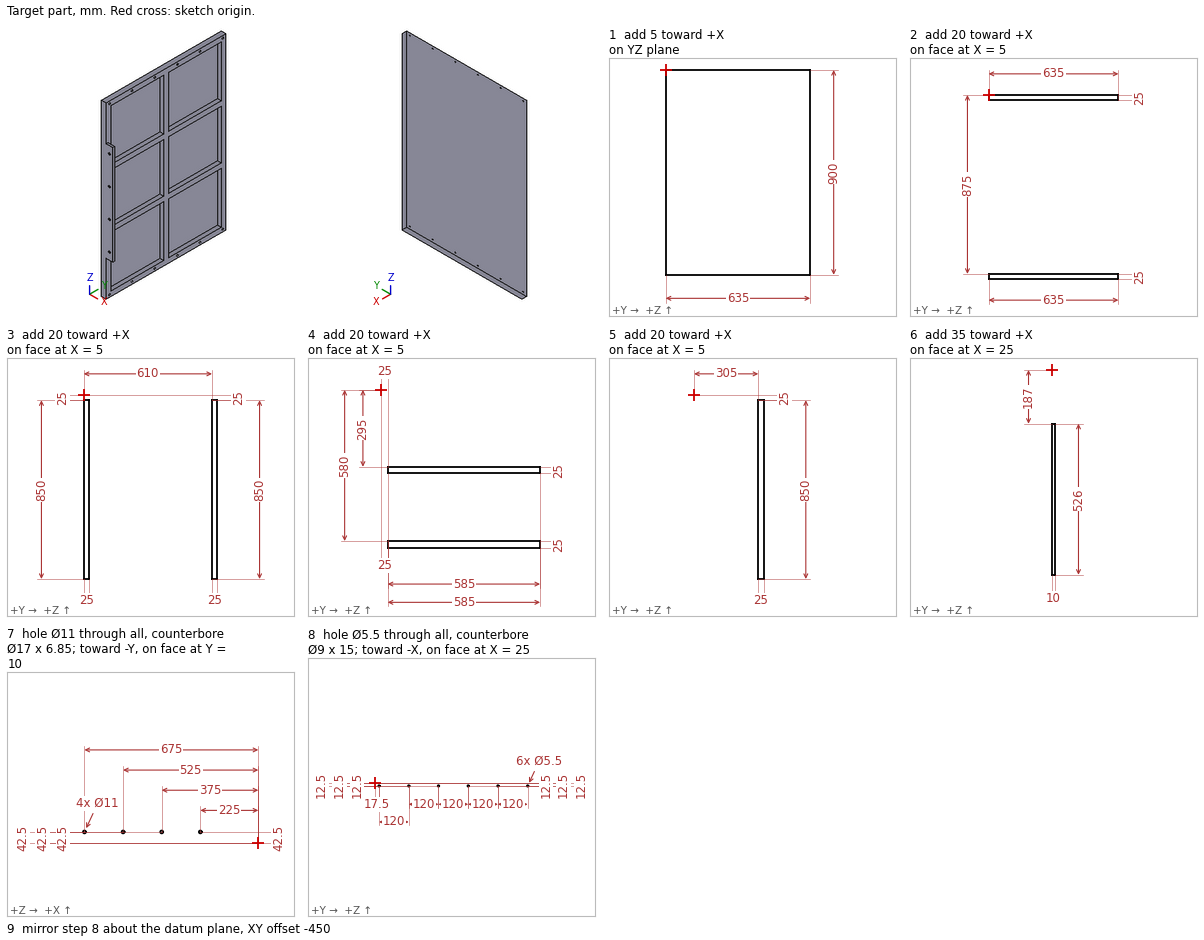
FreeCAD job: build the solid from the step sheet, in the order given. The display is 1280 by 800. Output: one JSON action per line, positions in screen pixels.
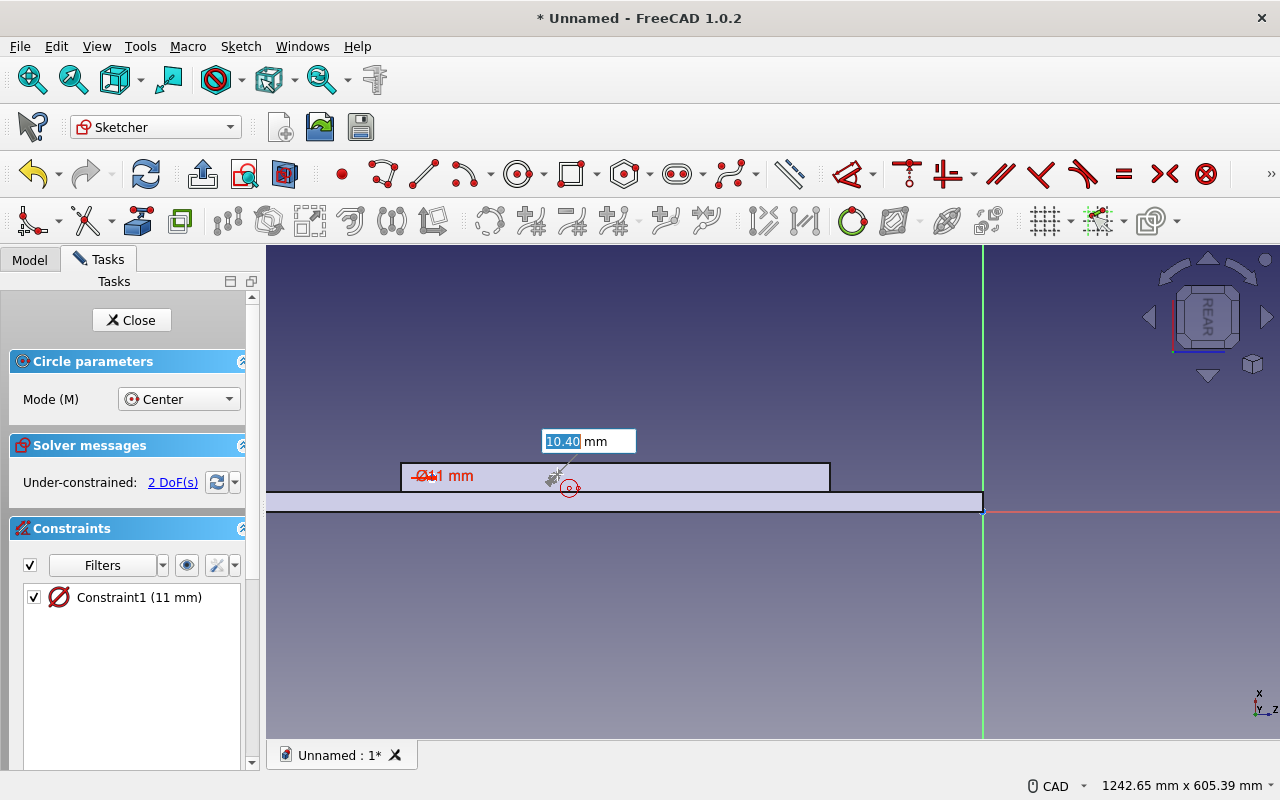
{"action": "type", "text": "11"}
{"action": "key", "text": "Return"}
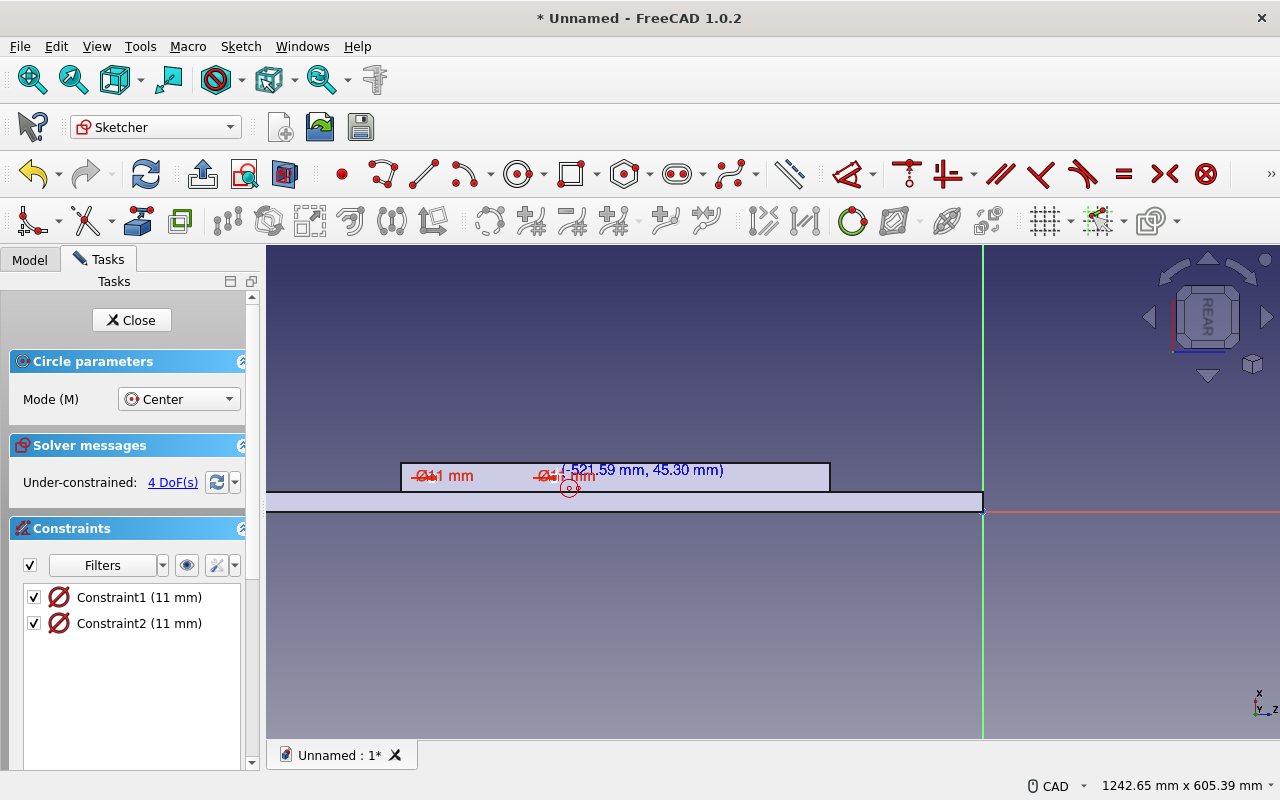
{"action": "scroll", "coordinate": [677, 477], "scroll_direction": "up", "scroll_amount": 9}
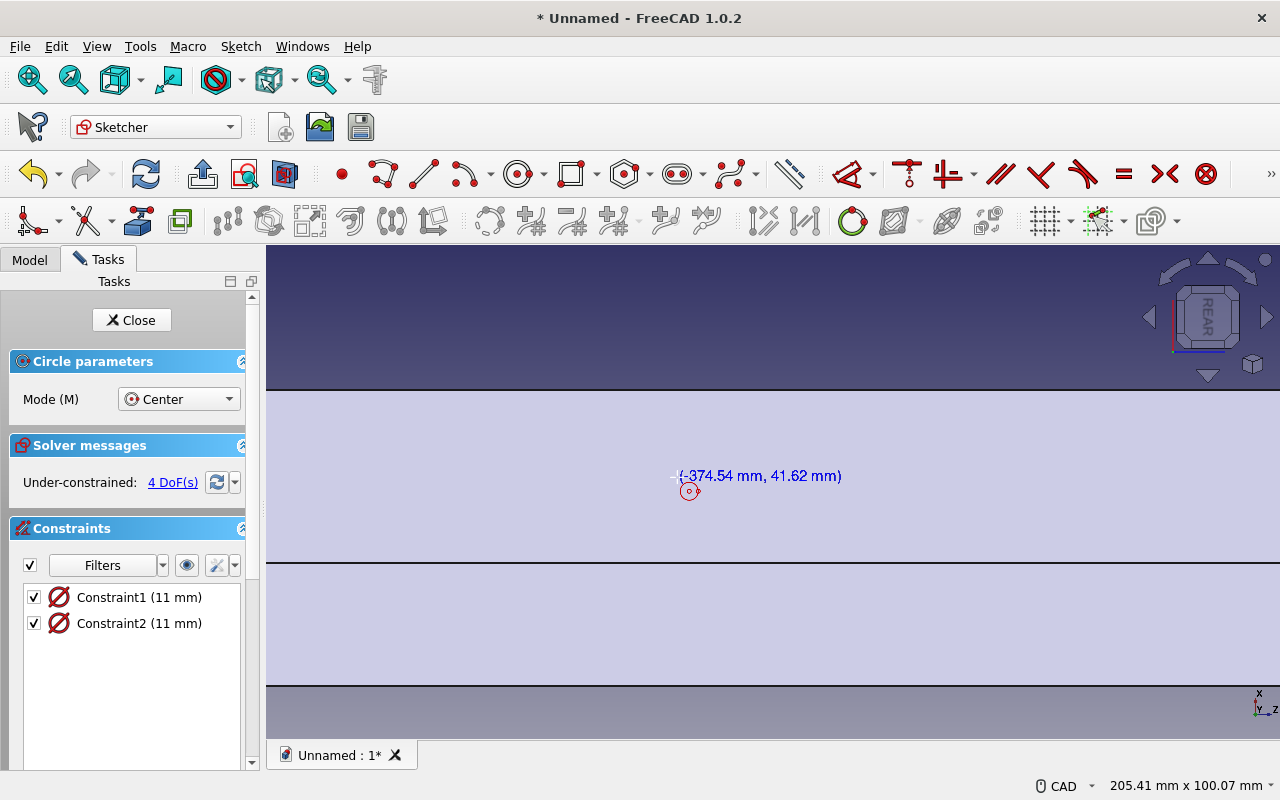
{"action": "scroll", "coordinate": [677, 477], "scroll_direction": "down", "scroll_amount": 9}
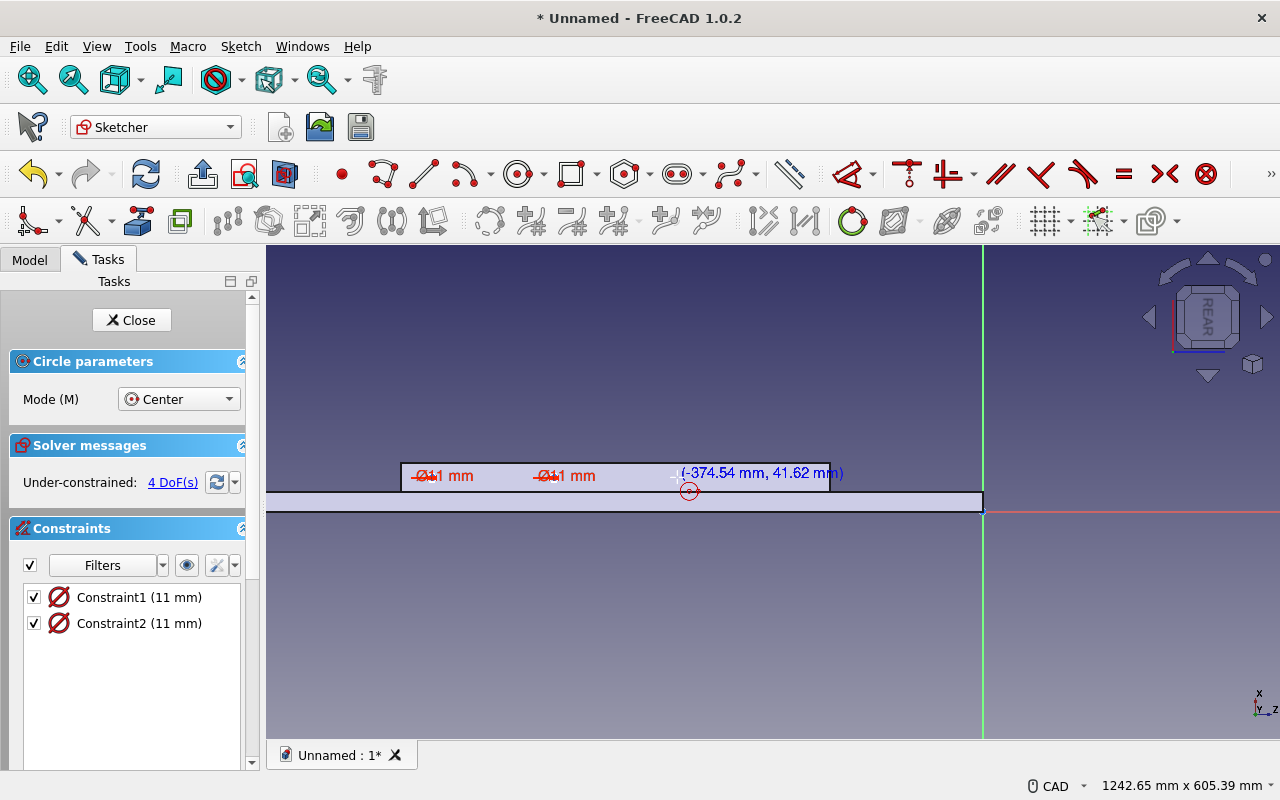
{"action": "left_click", "coordinate": [677, 477]}
{"action": "mouse_move", "coordinate": [680, 474]}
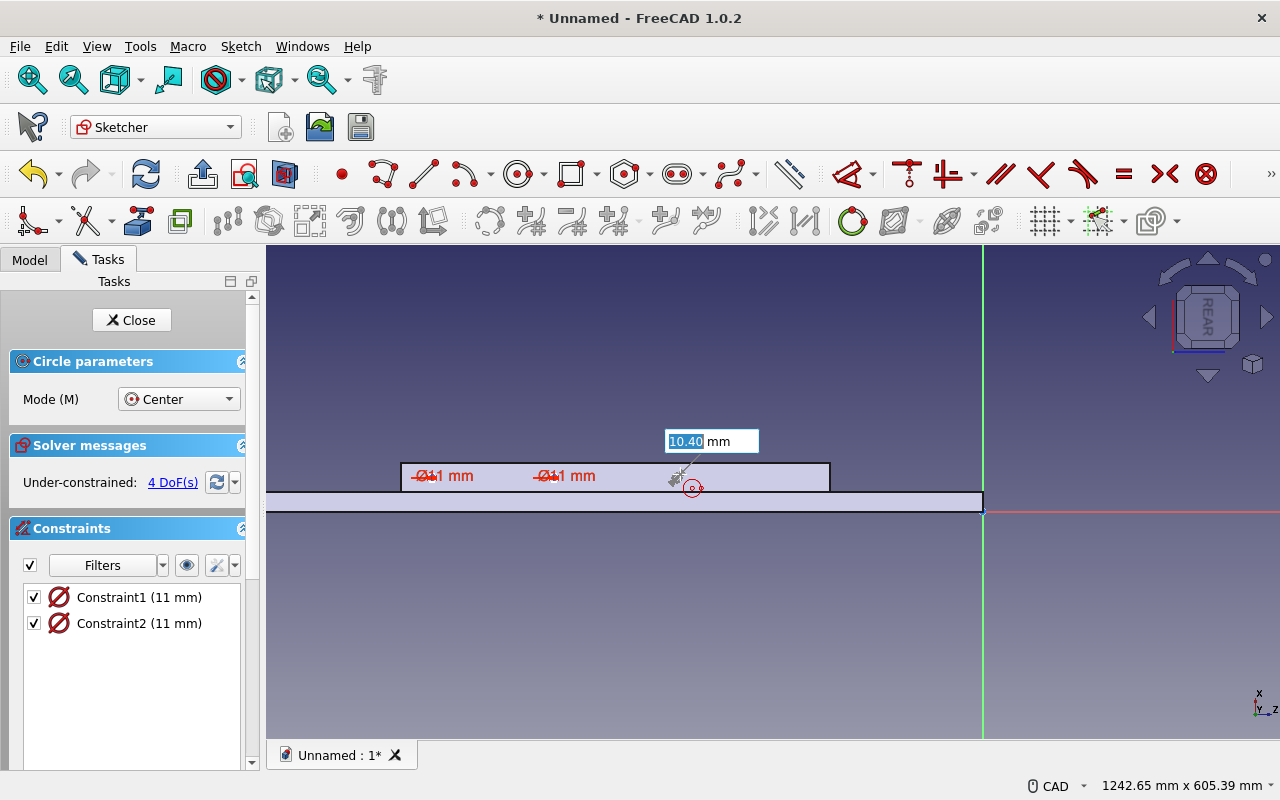
{"action": "type", "text": "11"}
{"action": "key", "text": "Return"}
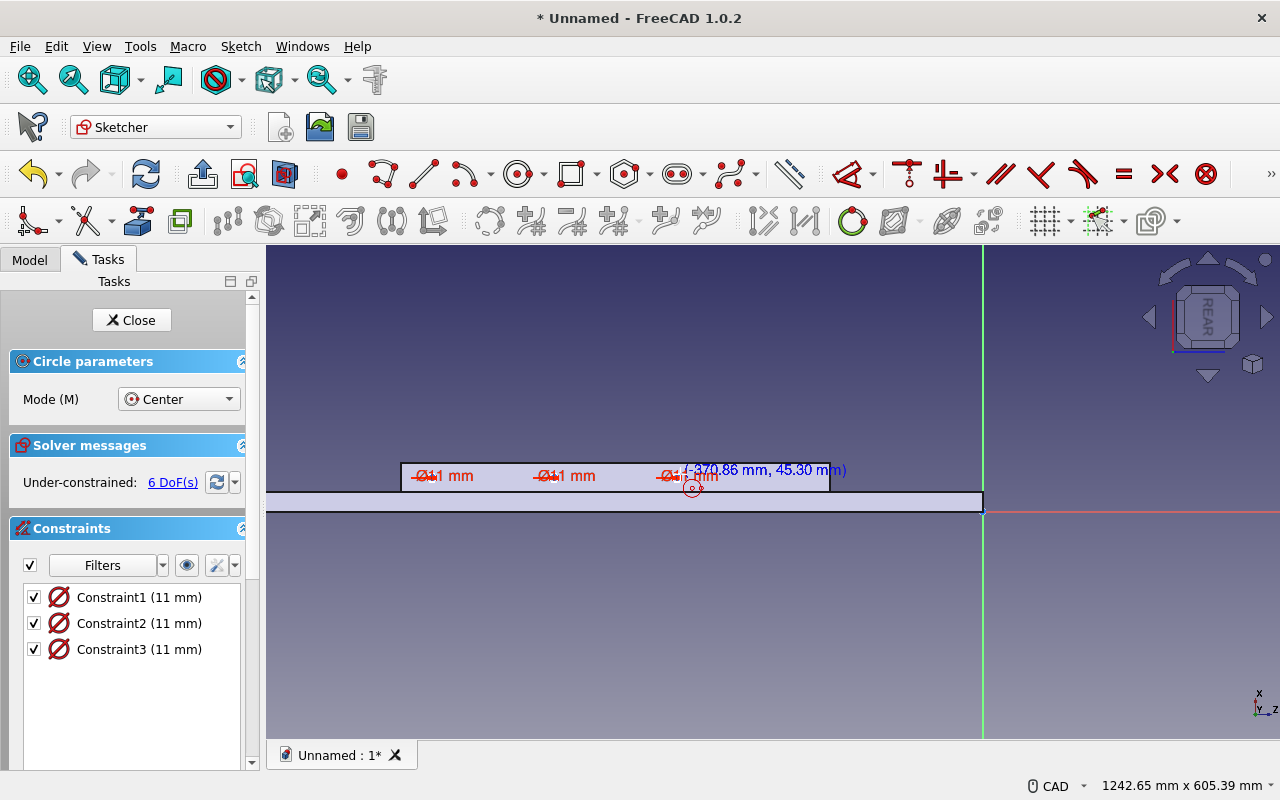
{"action": "scroll", "coordinate": [799, 477], "scroll_direction": "up", "scroll_amount": 9}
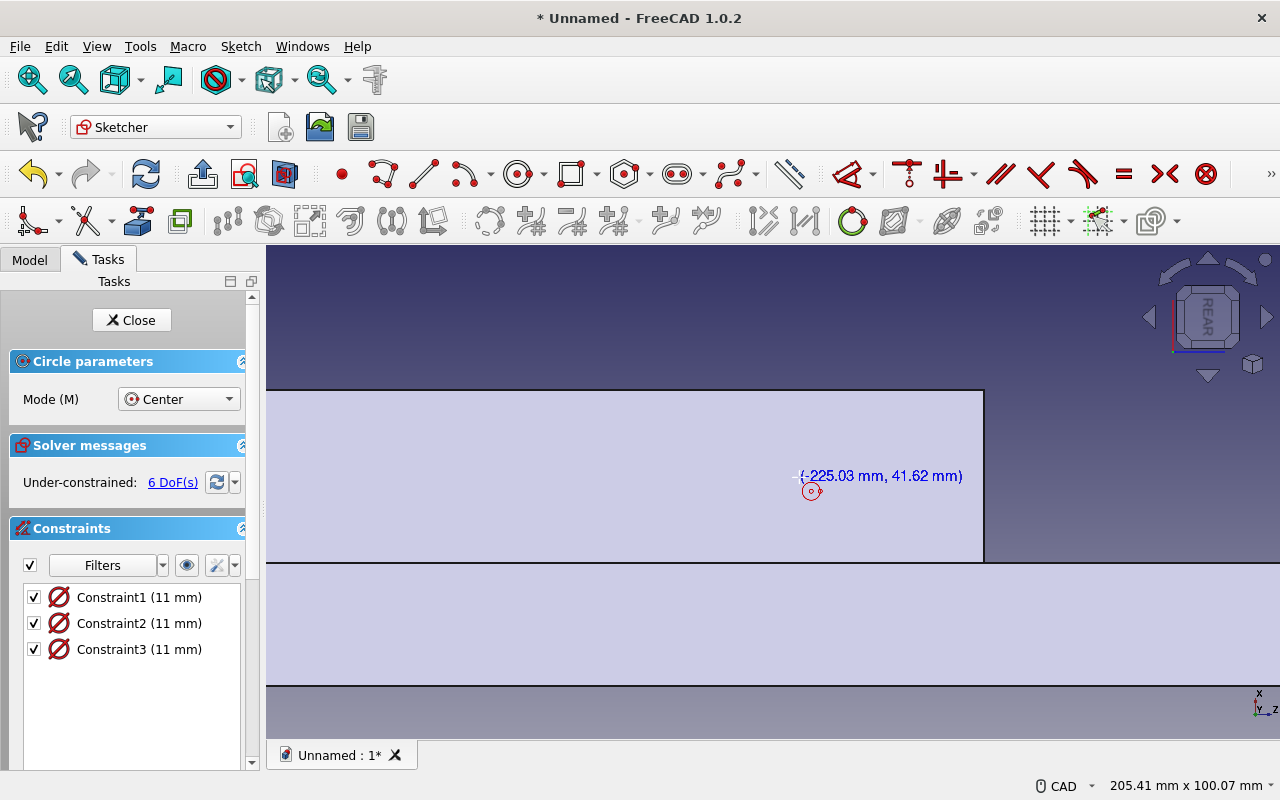
{"action": "scroll", "coordinate": [799, 477], "scroll_direction": "down", "scroll_amount": 9}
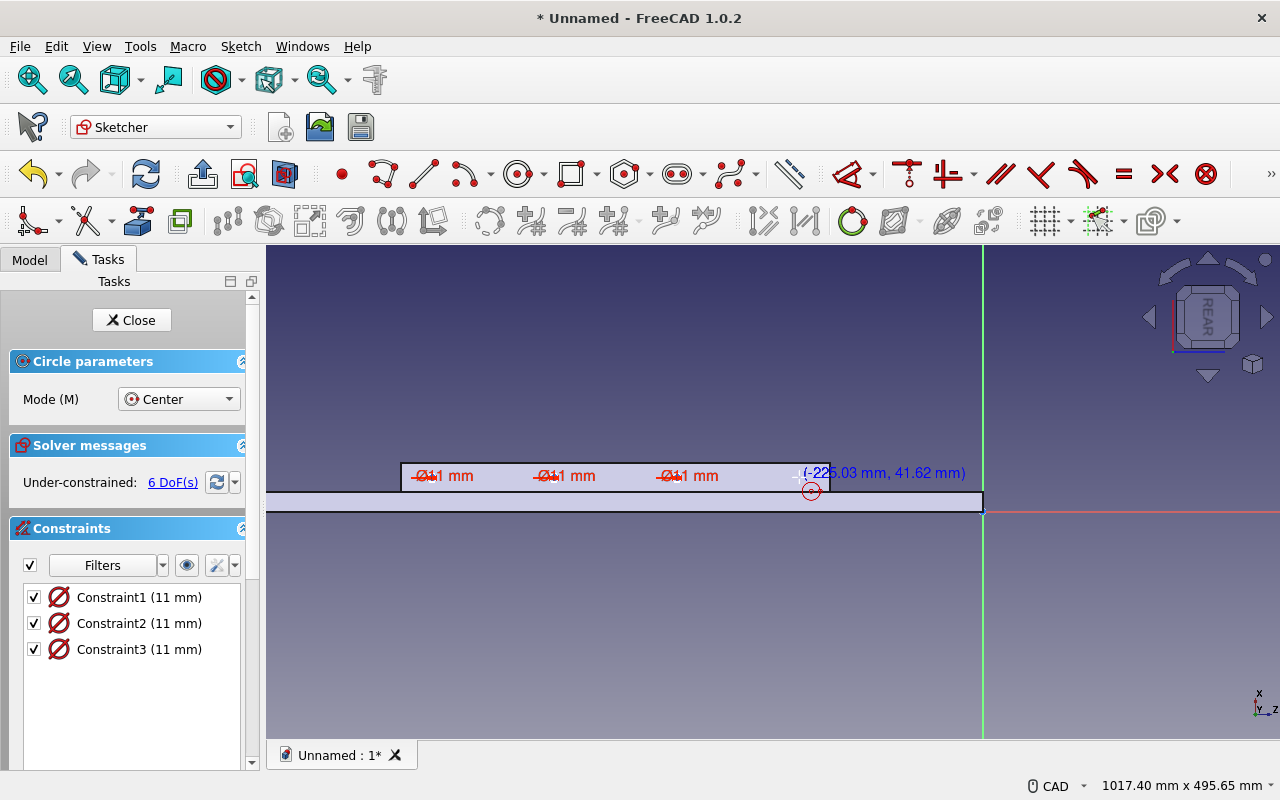
{"action": "left_click", "coordinate": [799, 477]}
{"action": "mouse_move", "coordinate": [802, 474]}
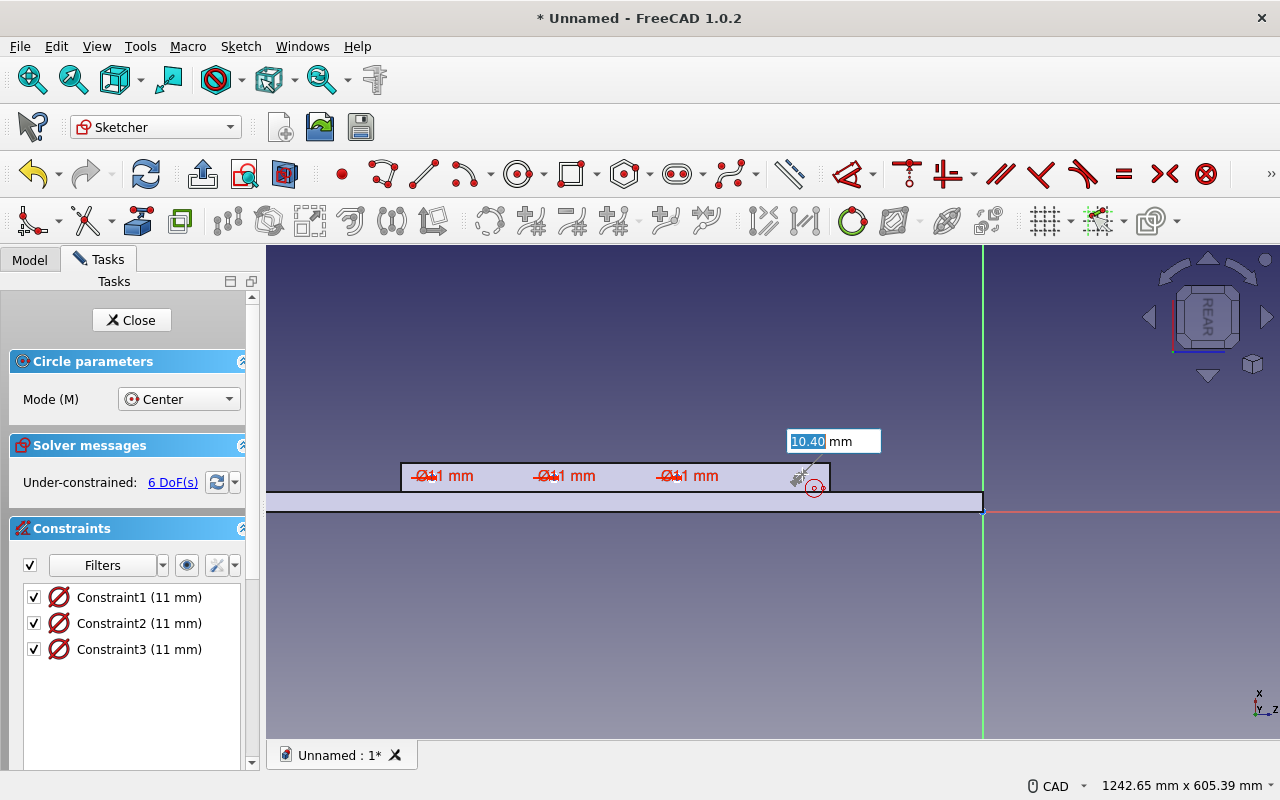
{"action": "type", "text": "11"}
{"action": "key", "text": "Return"}
{"action": "key", "text": "Escape"}